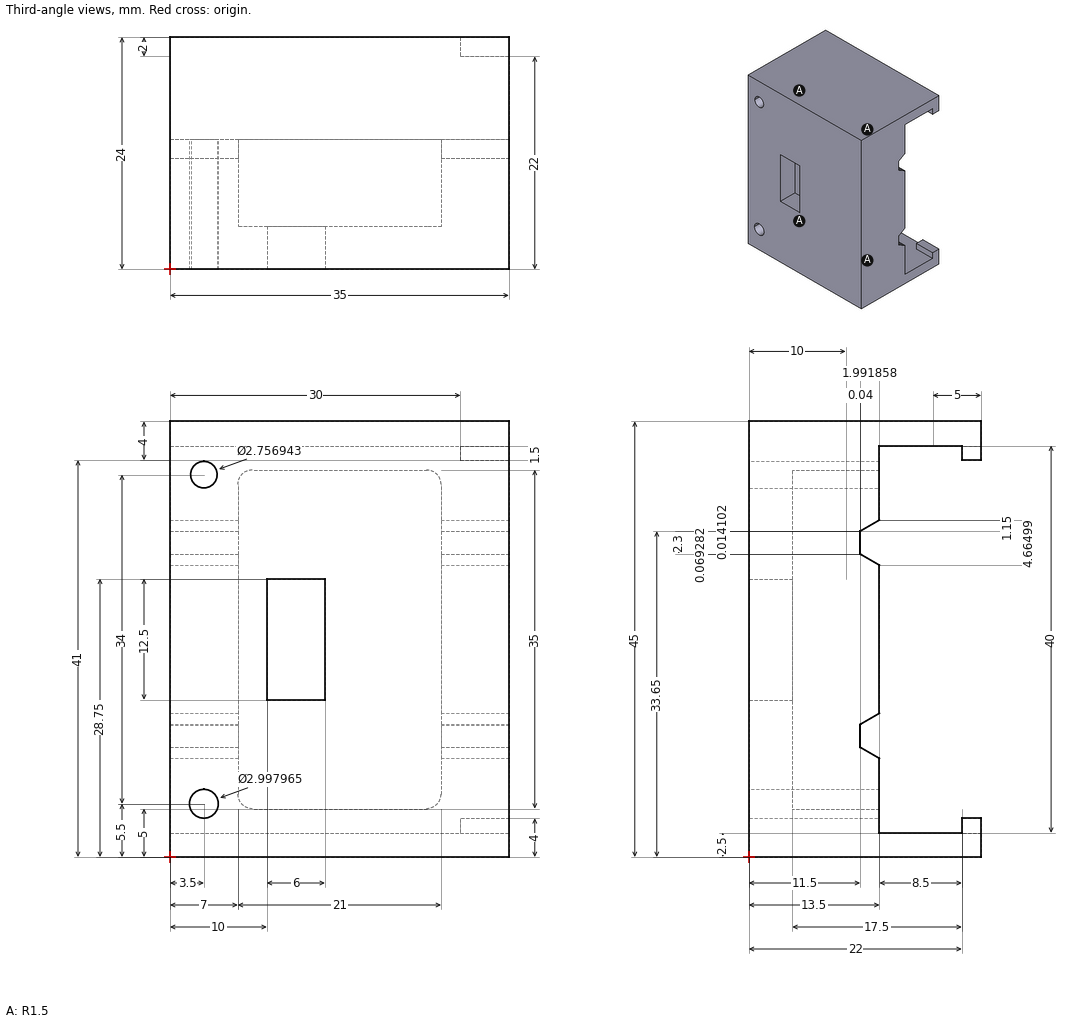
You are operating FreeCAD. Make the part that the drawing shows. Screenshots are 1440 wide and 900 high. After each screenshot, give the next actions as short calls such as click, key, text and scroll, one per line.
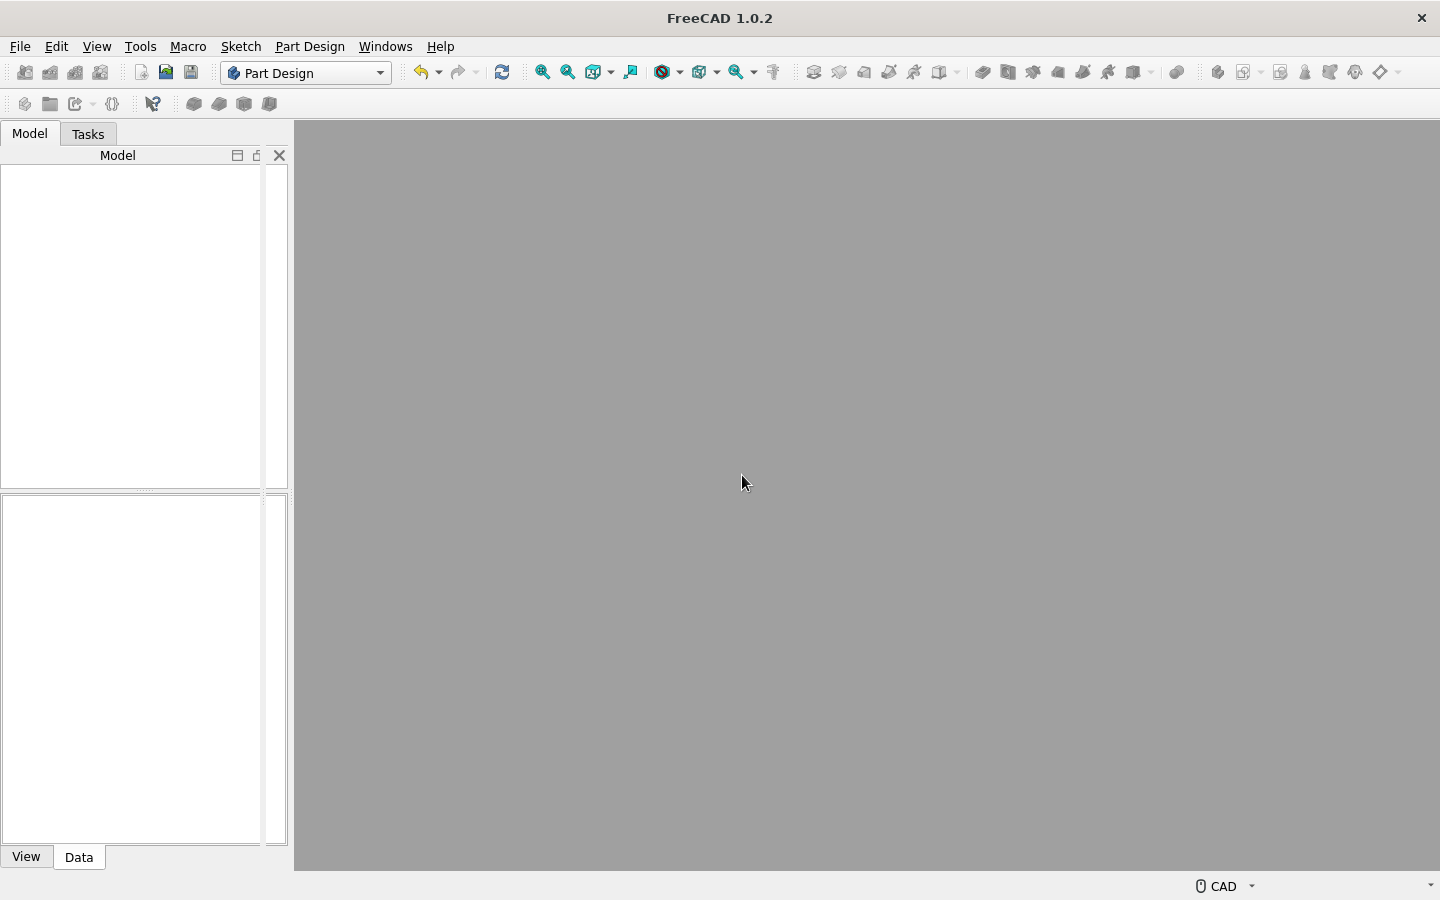
key(ctrl+n)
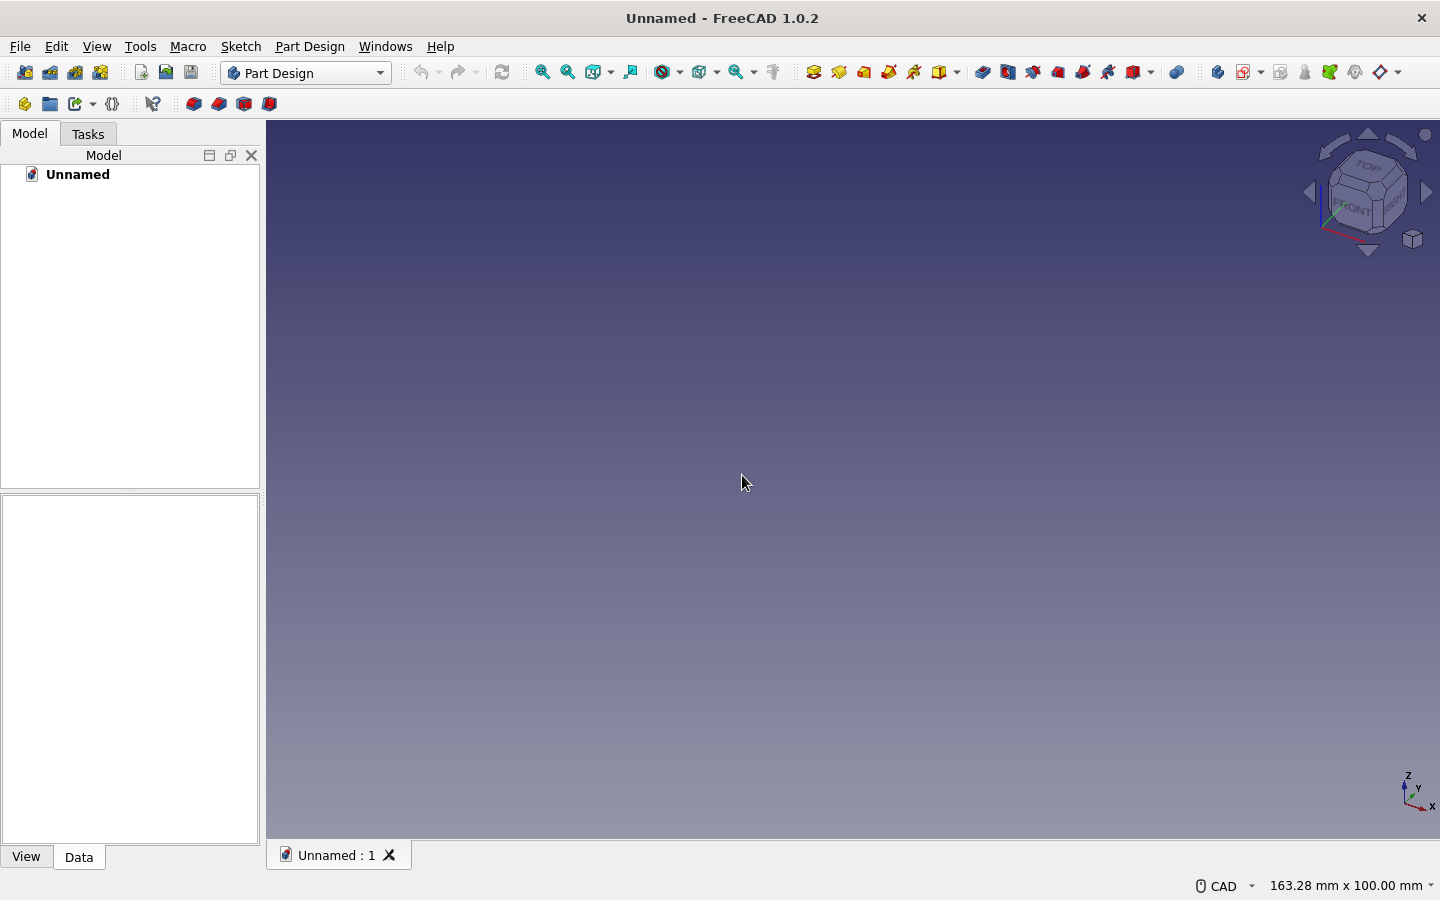
click(1242, 72)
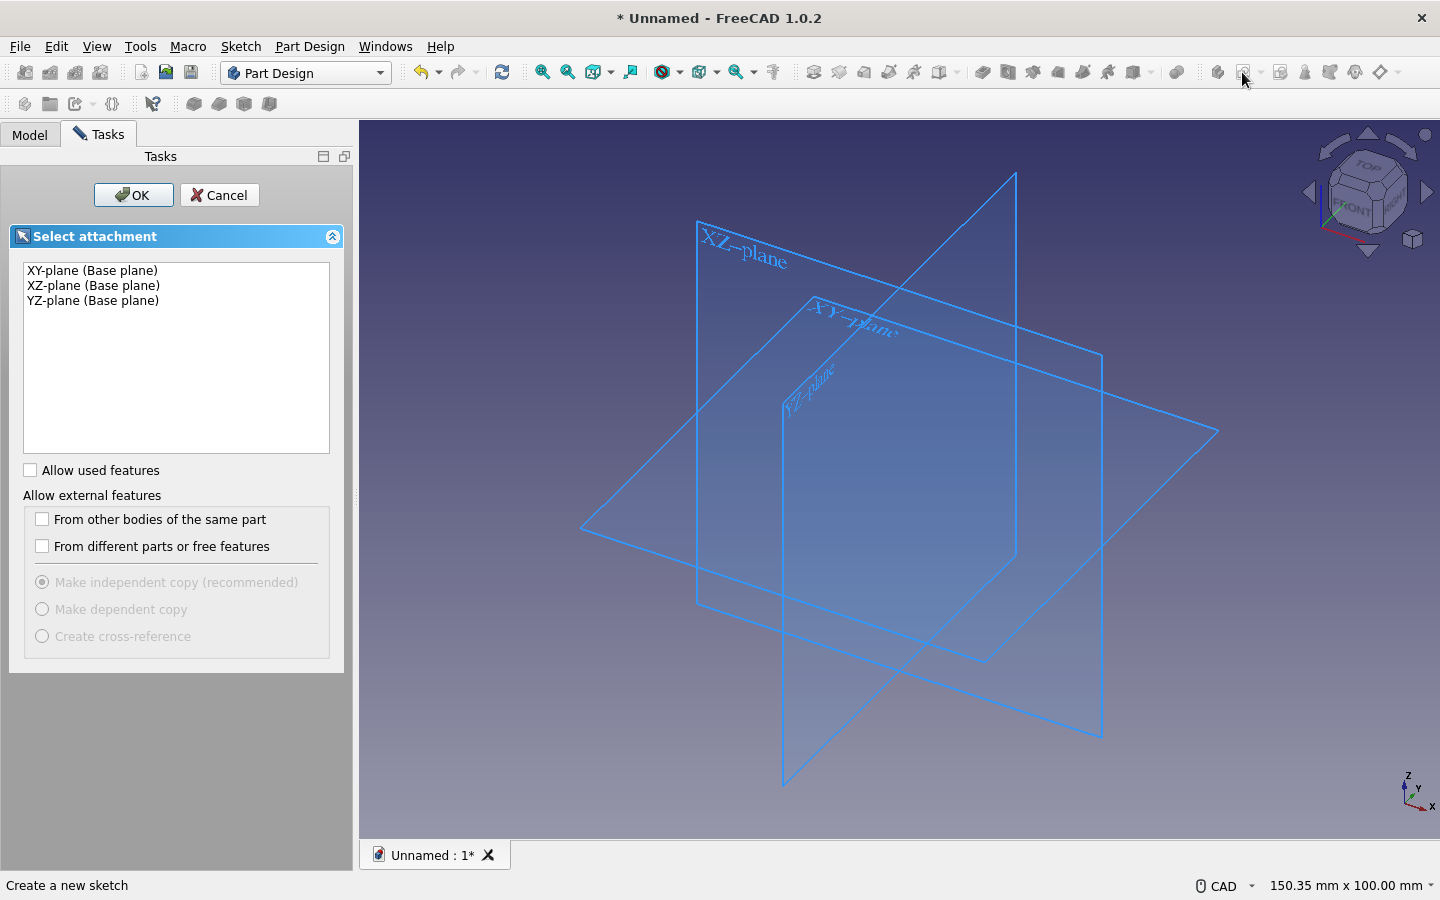
click(84, 270)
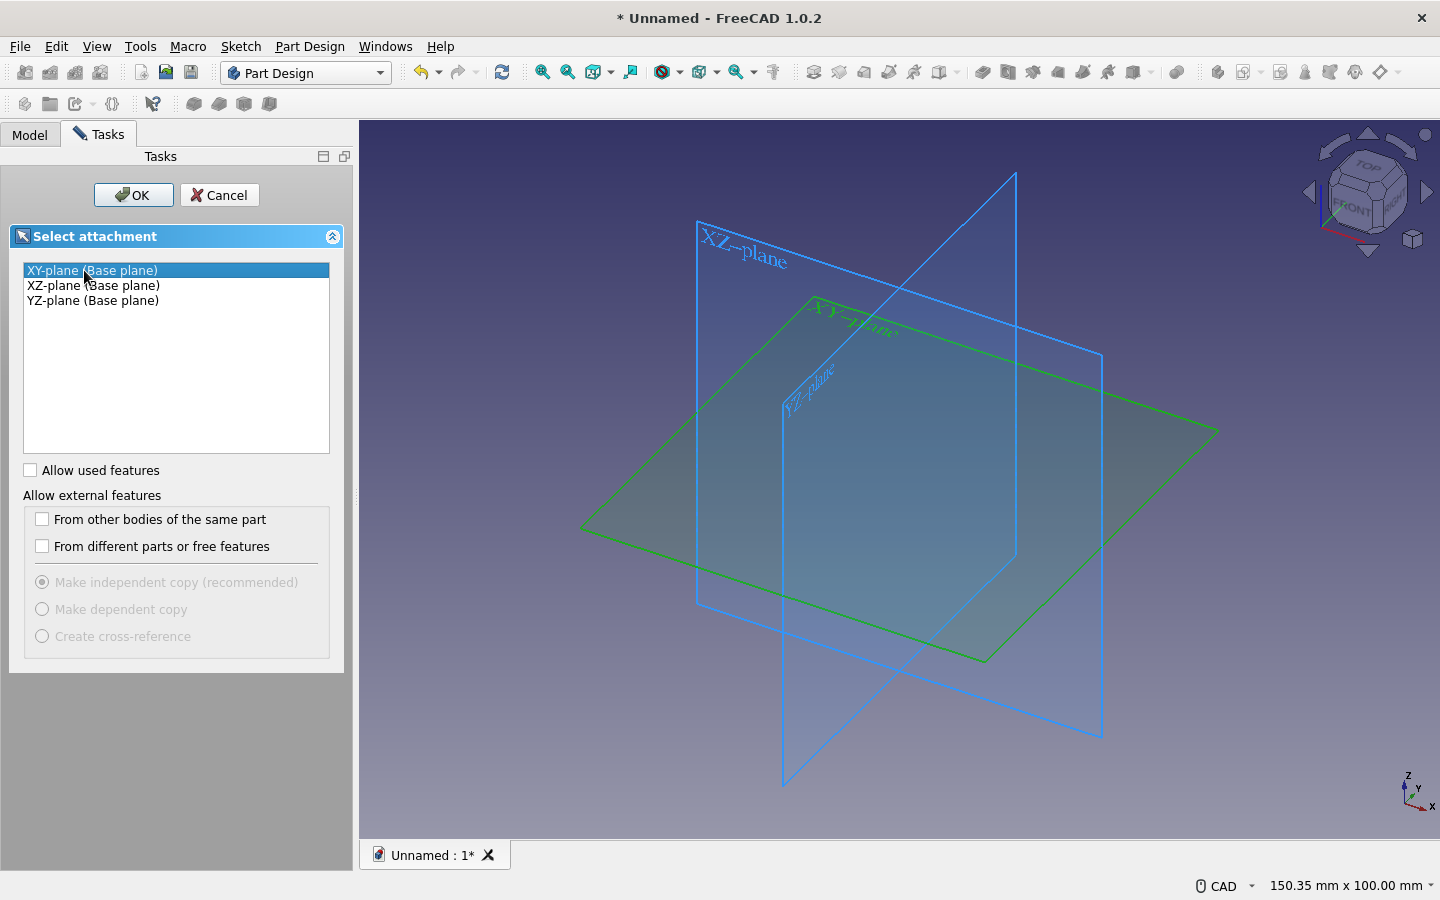
click(134, 195)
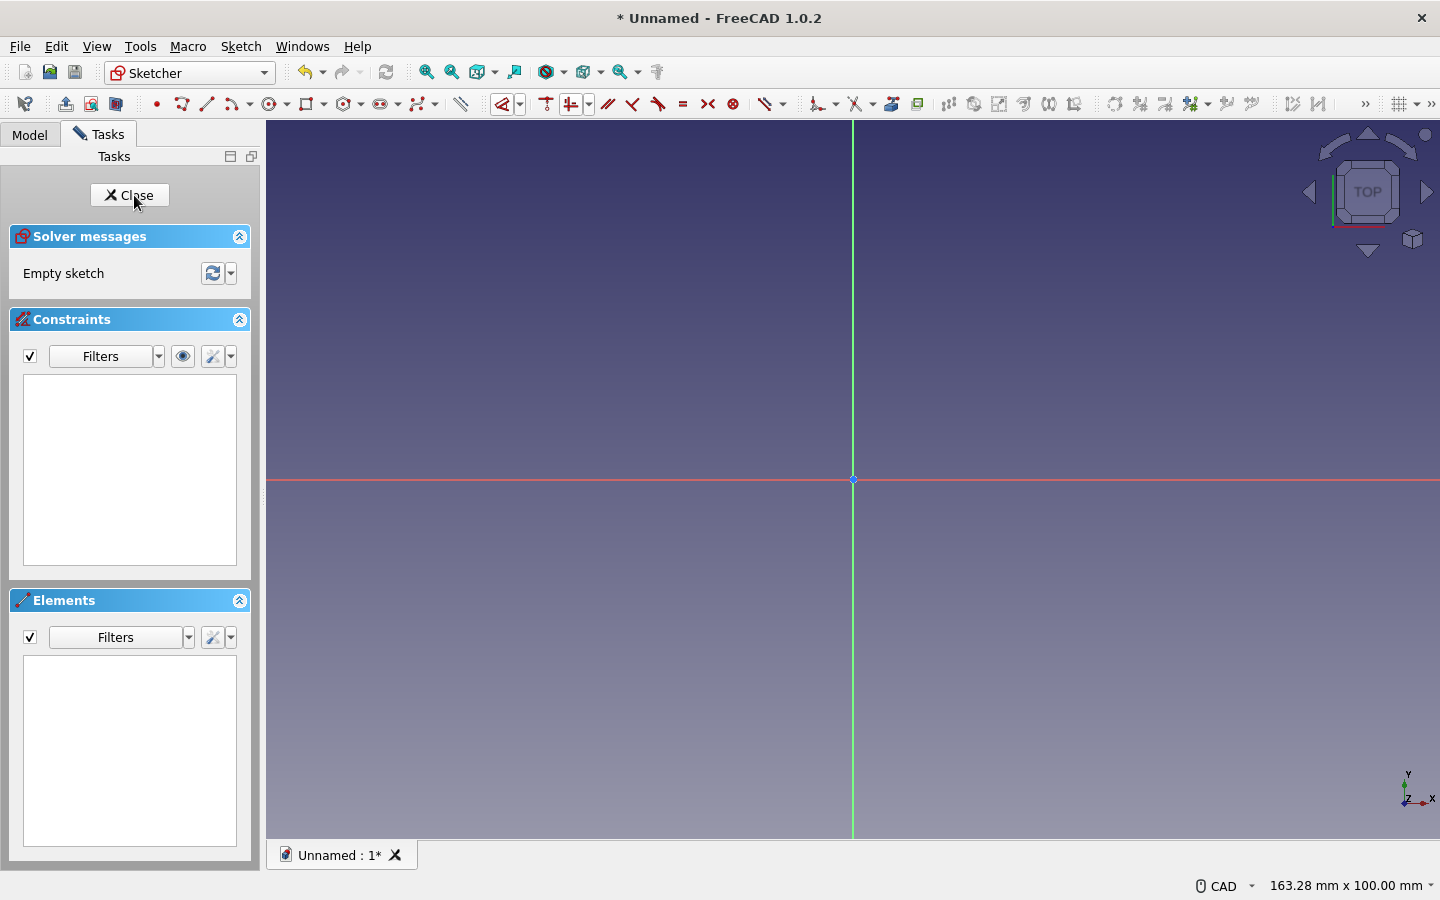
scroll(1092, 354, up, 5)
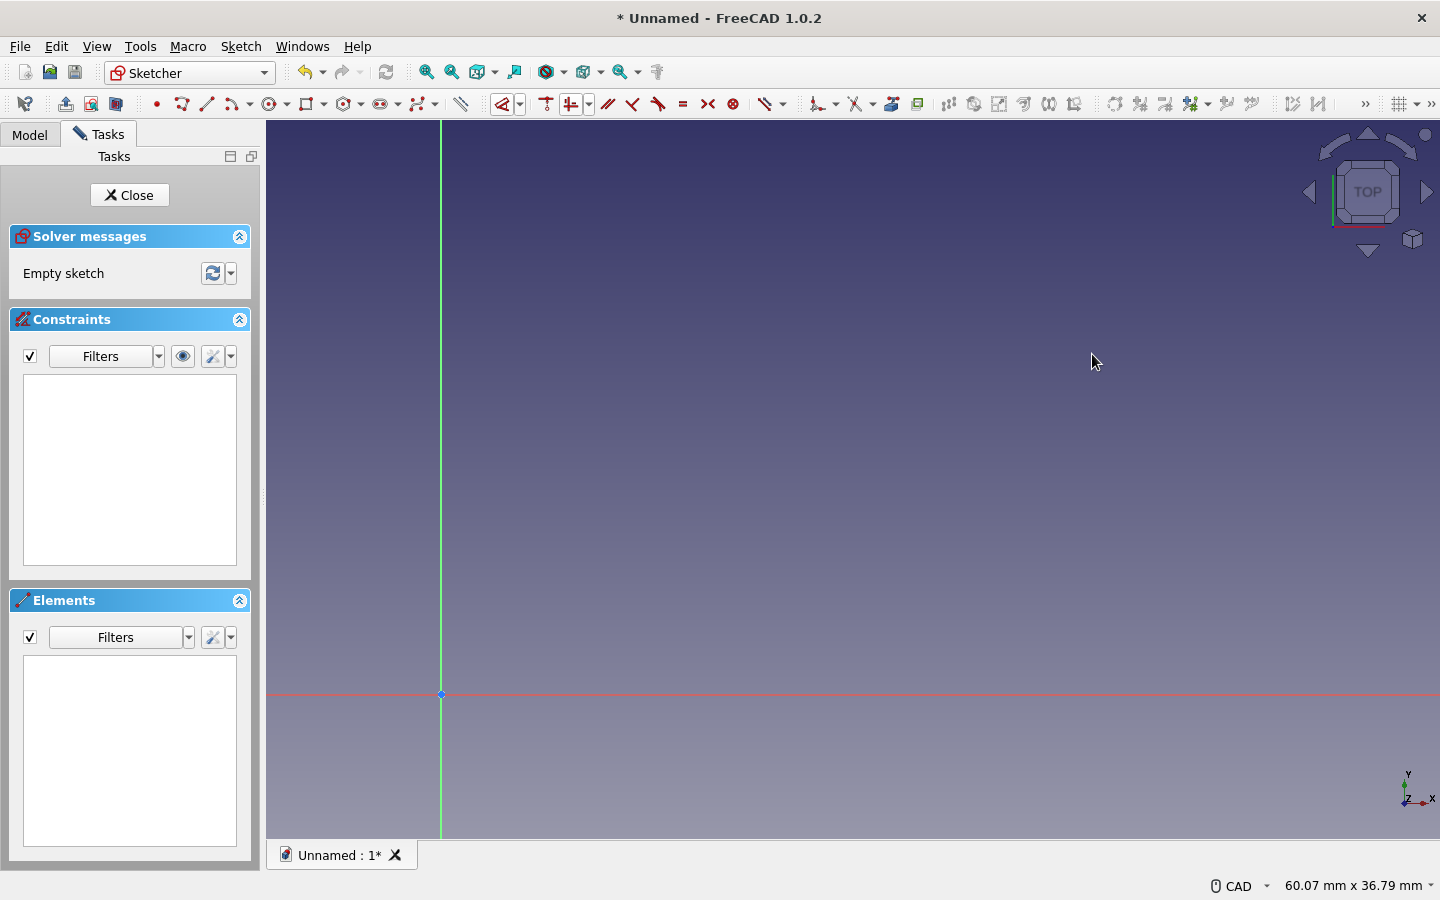
click(306, 104)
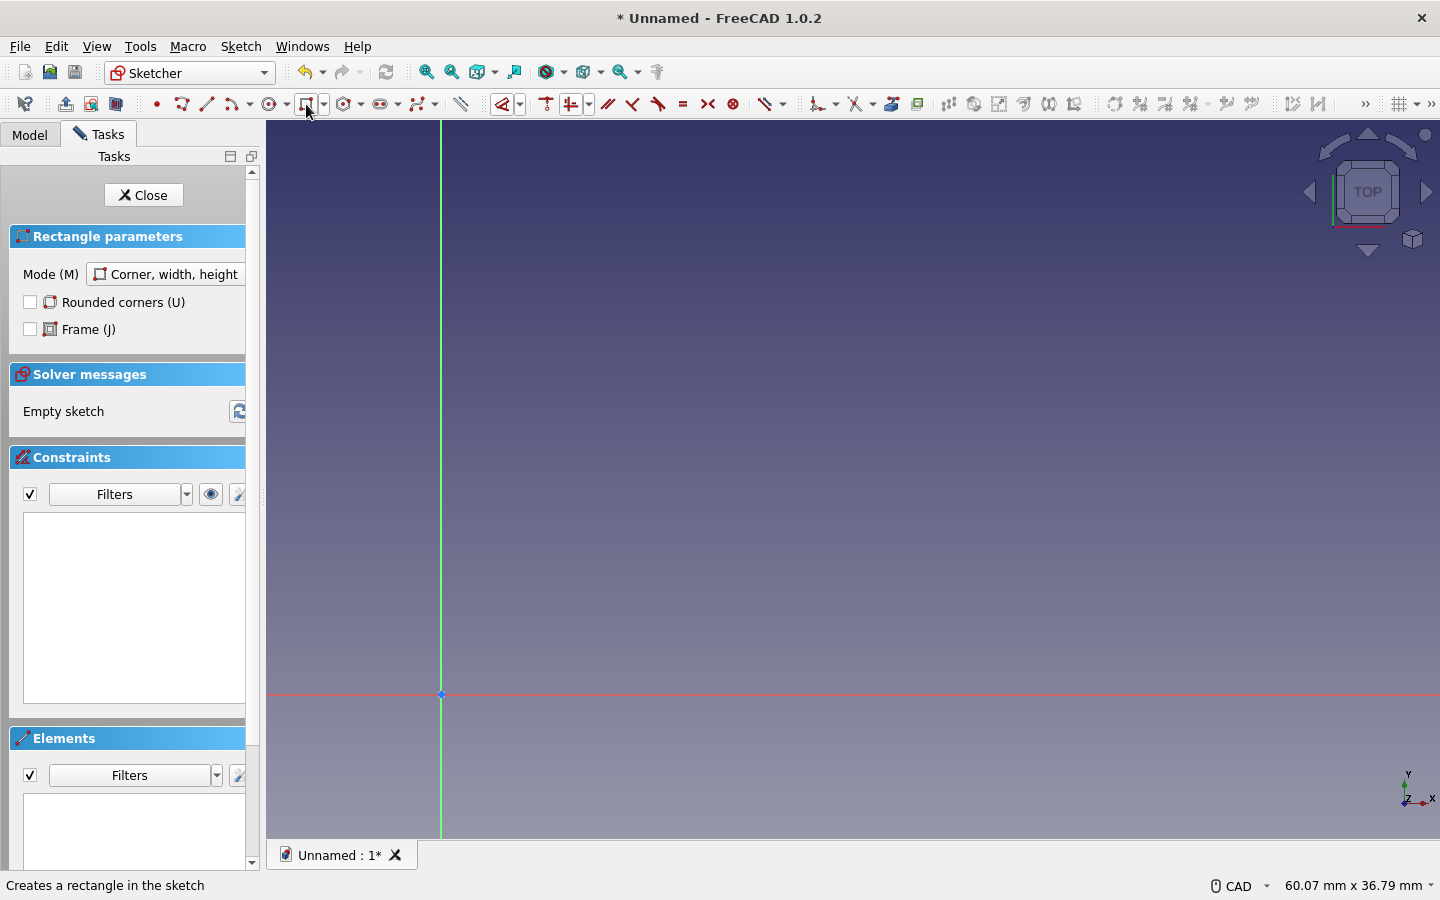
click(441, 695)
click(1125, 265)
key(Escape)